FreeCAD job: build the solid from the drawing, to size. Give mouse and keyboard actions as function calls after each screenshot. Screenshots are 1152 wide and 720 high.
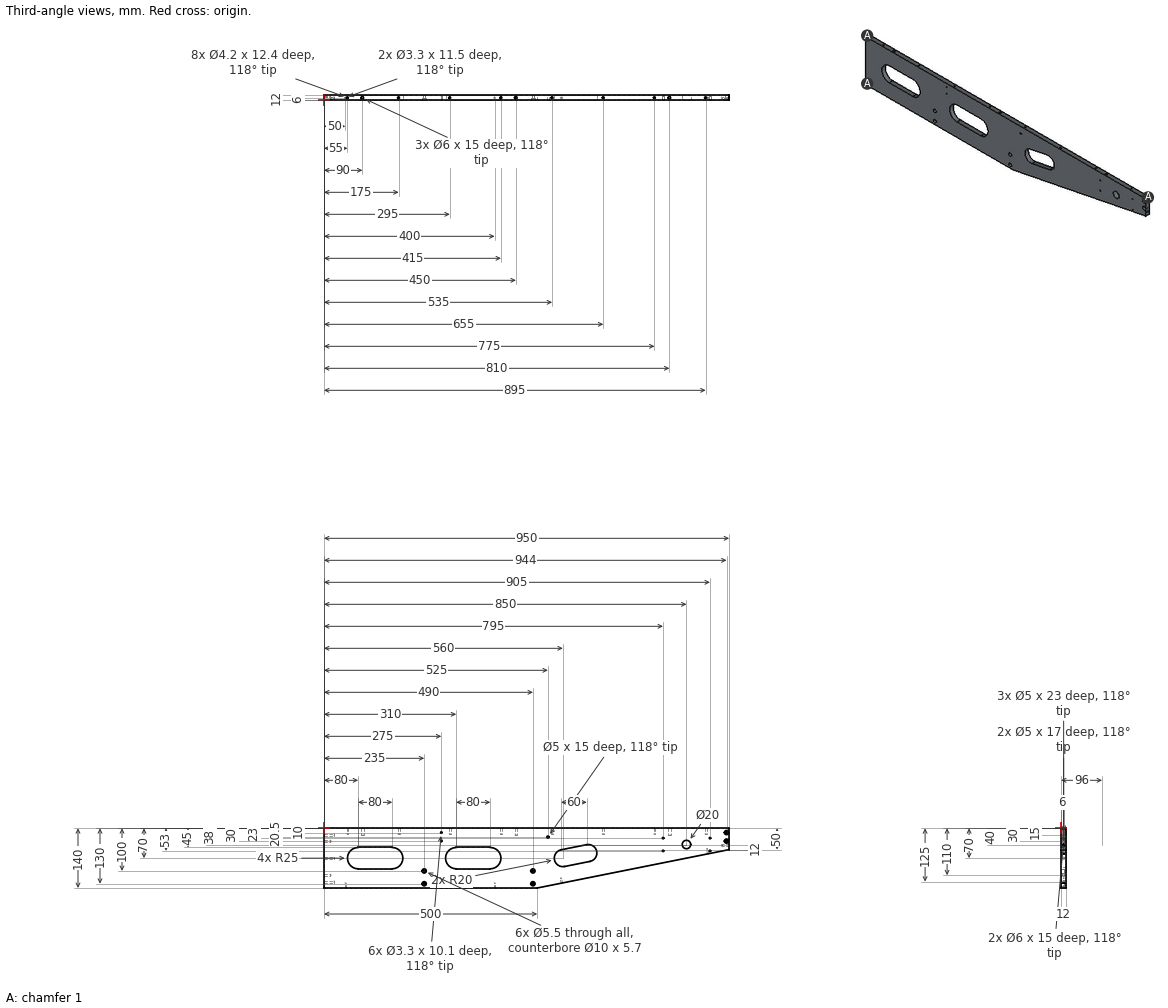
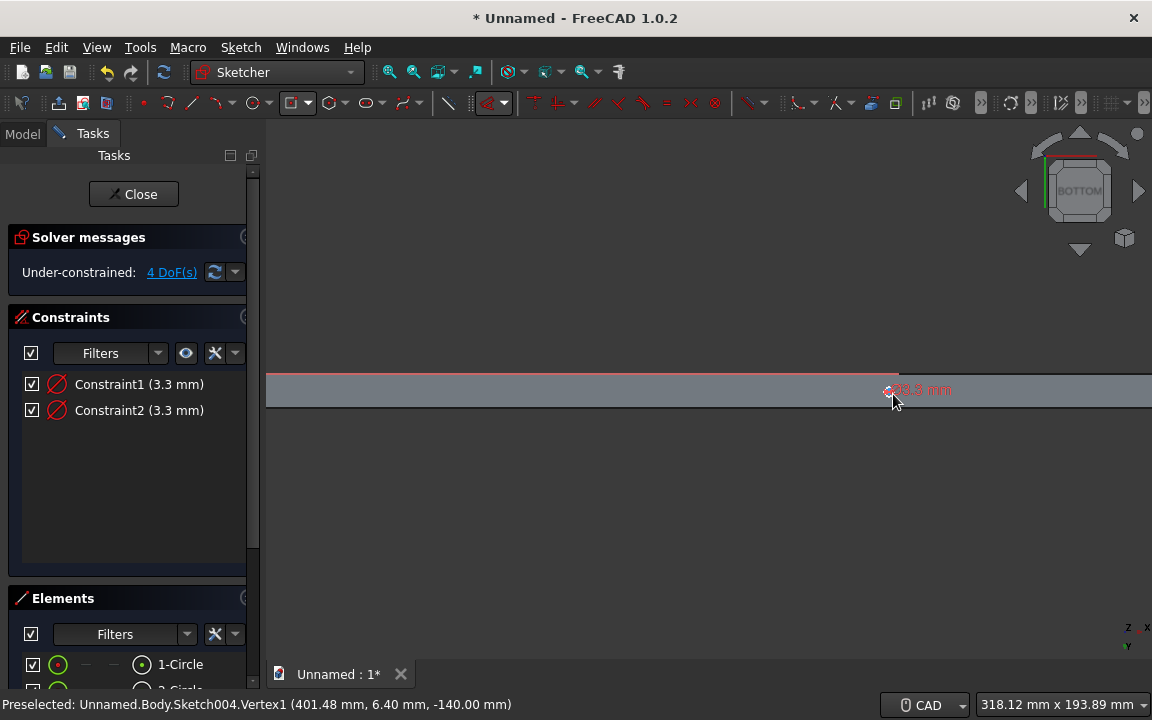
scroll(890, 392, down, 4)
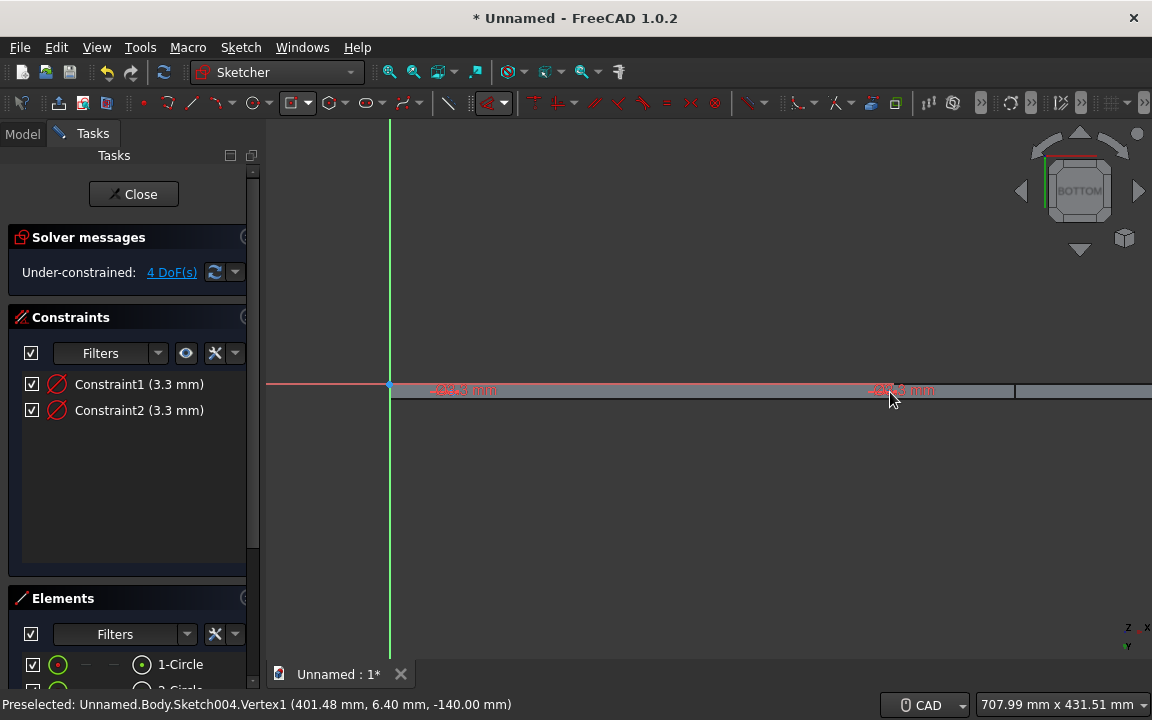
click(452, 392)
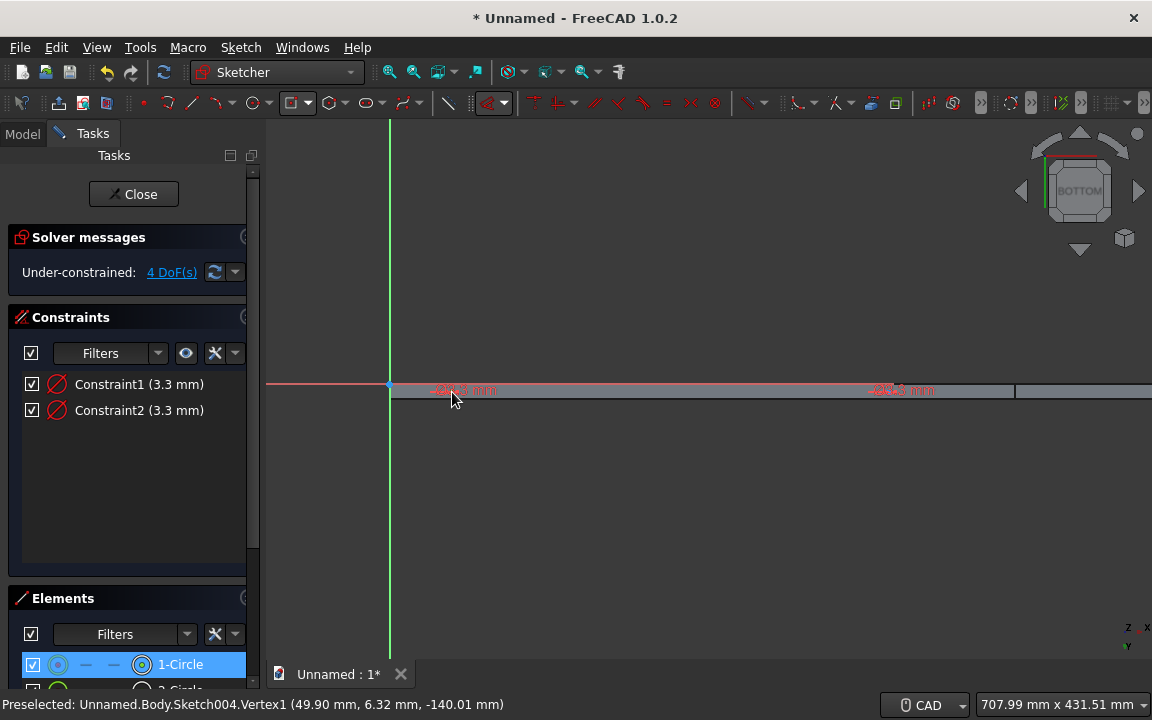
click(890, 392)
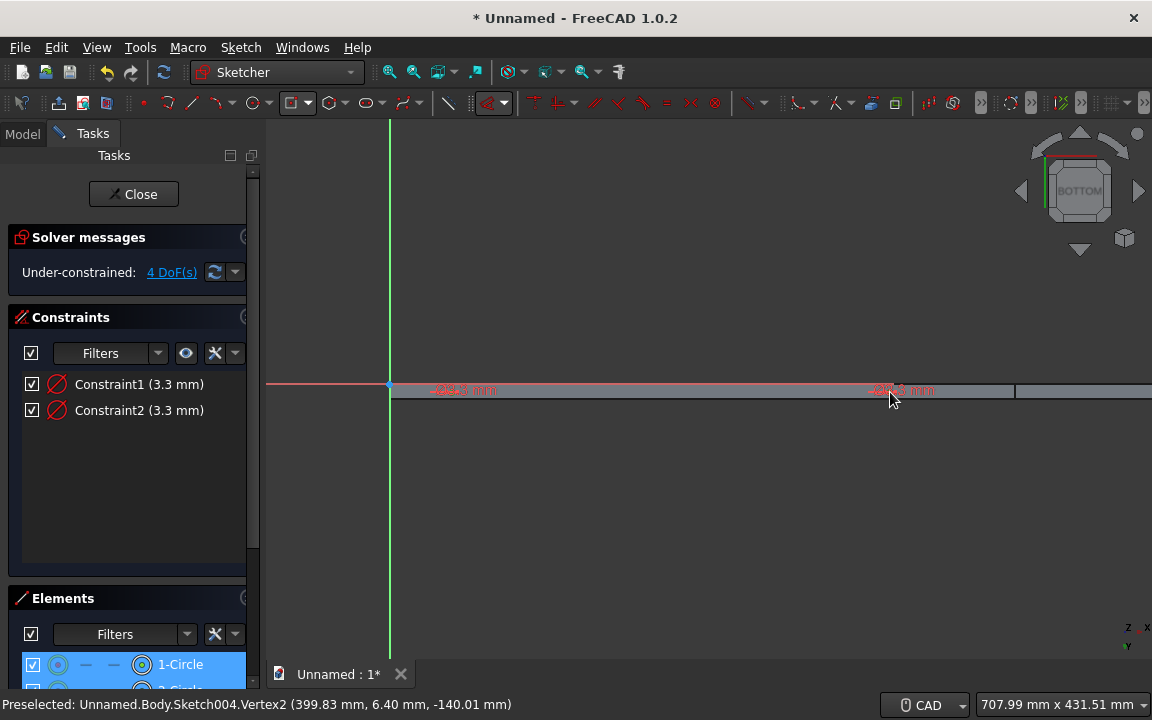
key(h)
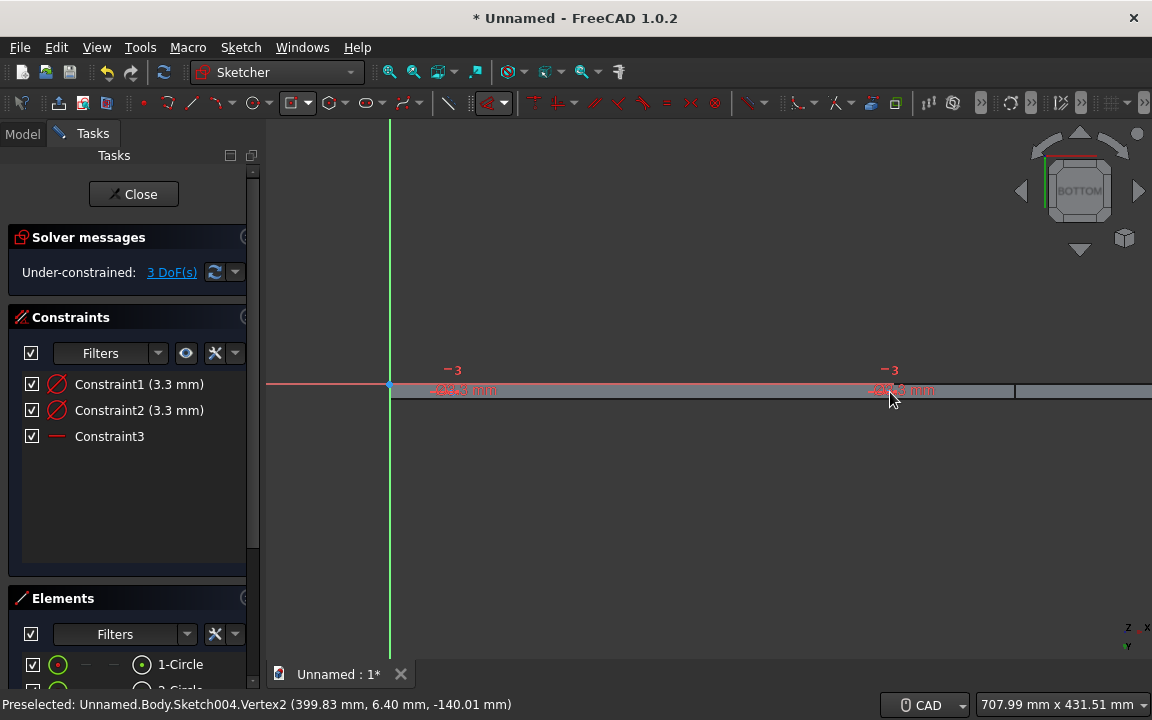
scroll(452, 392, up, 9)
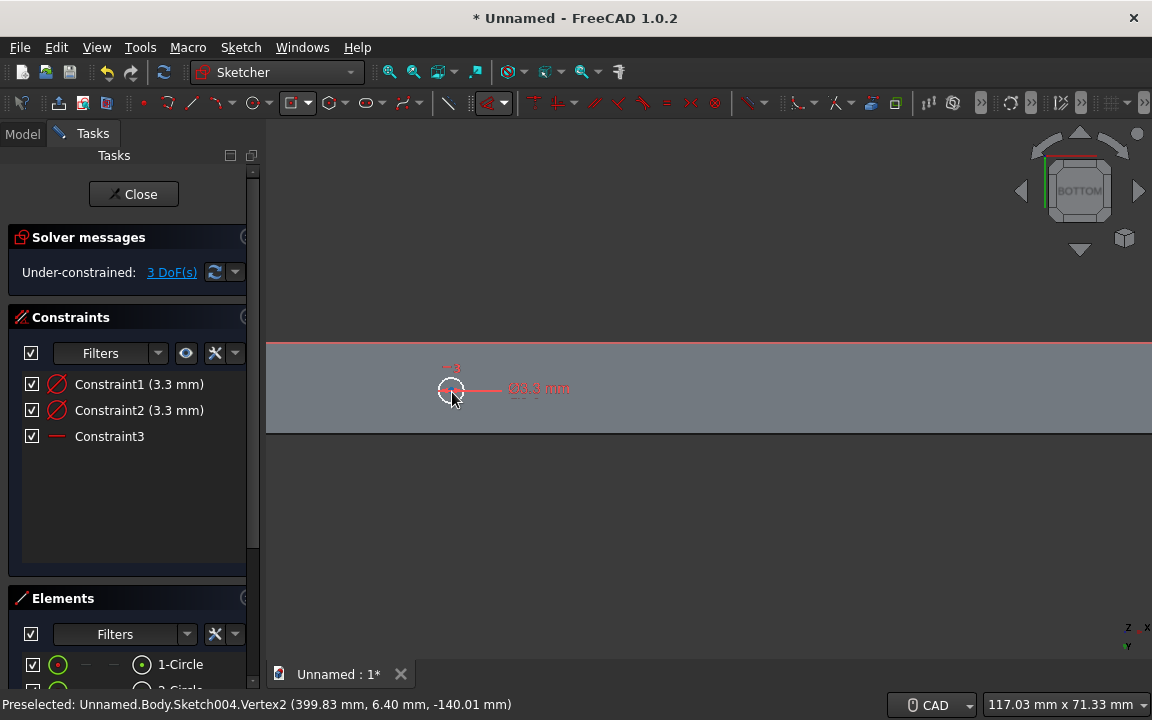
click(451, 391)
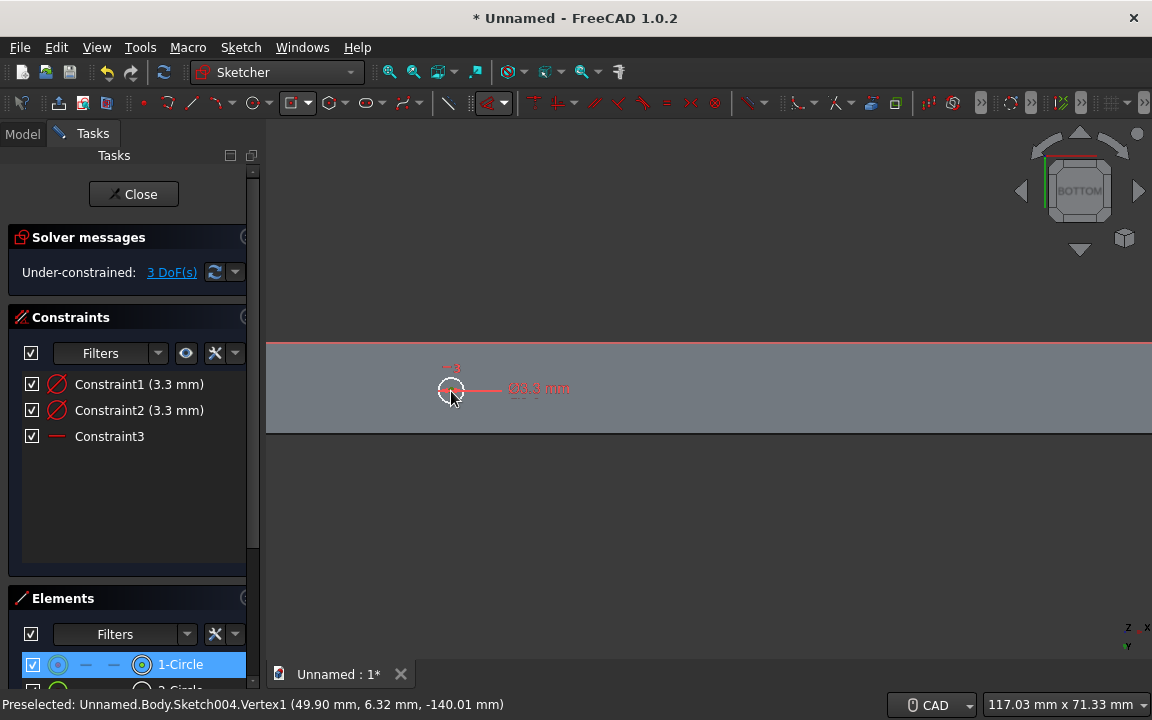
key(i)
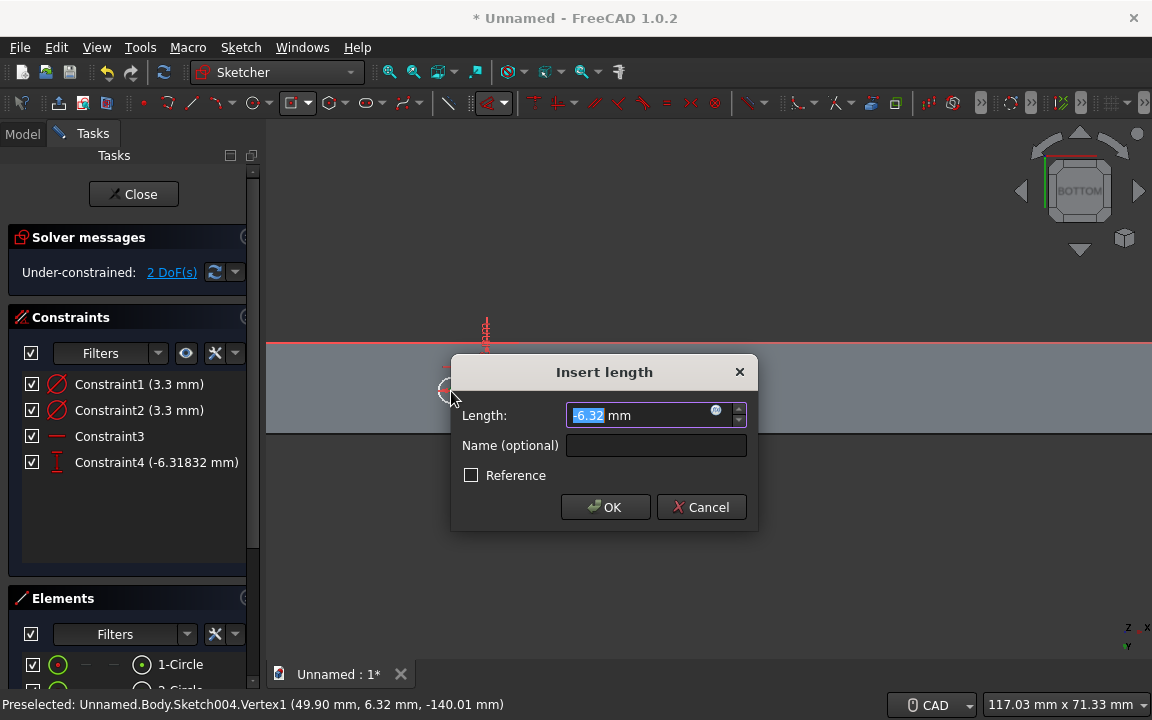
text(-6)
key(Return)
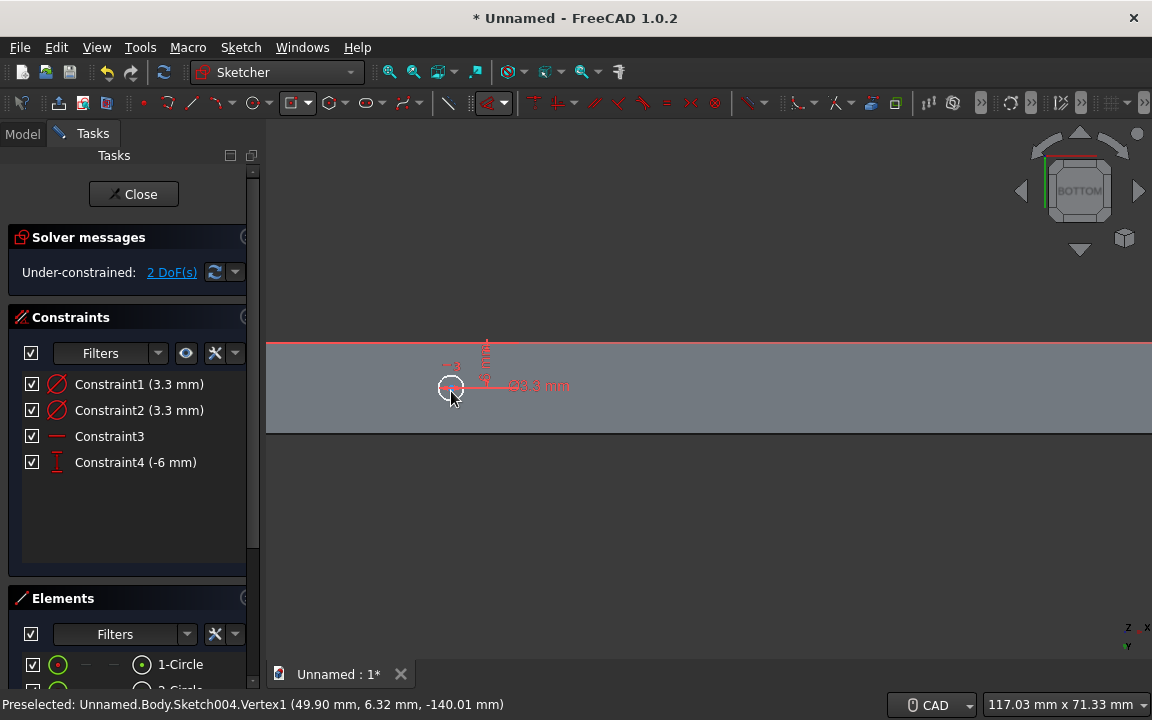
scroll(452, 392, down, 9)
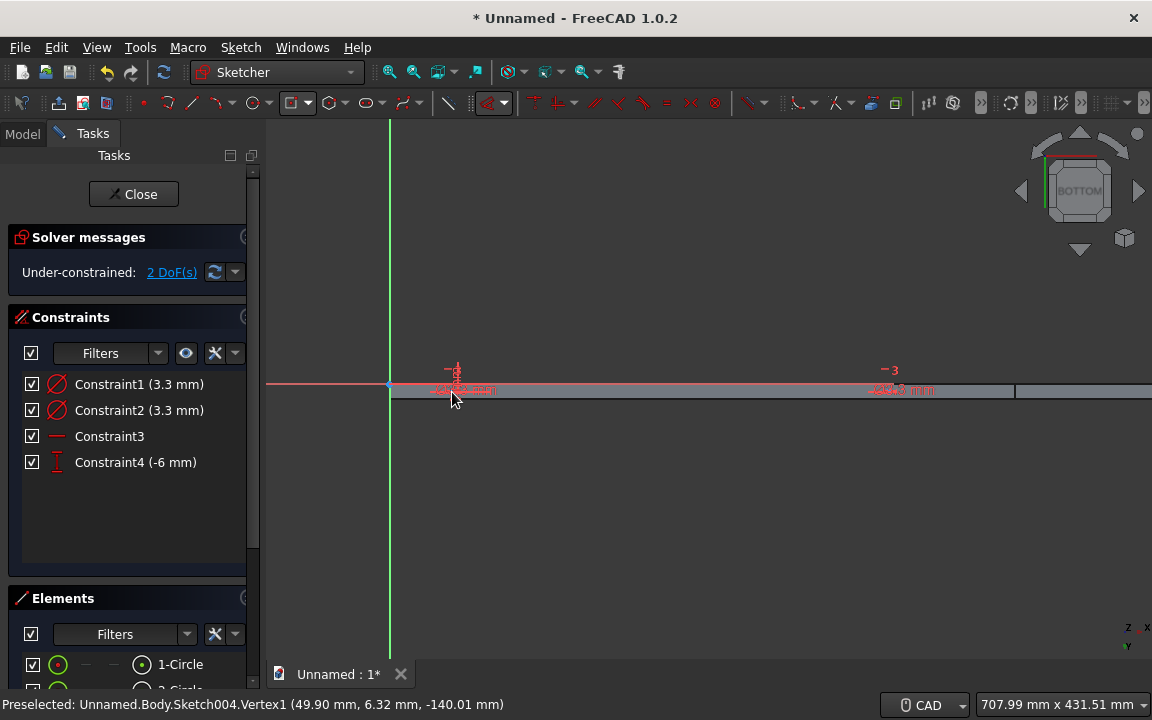
click(452, 392)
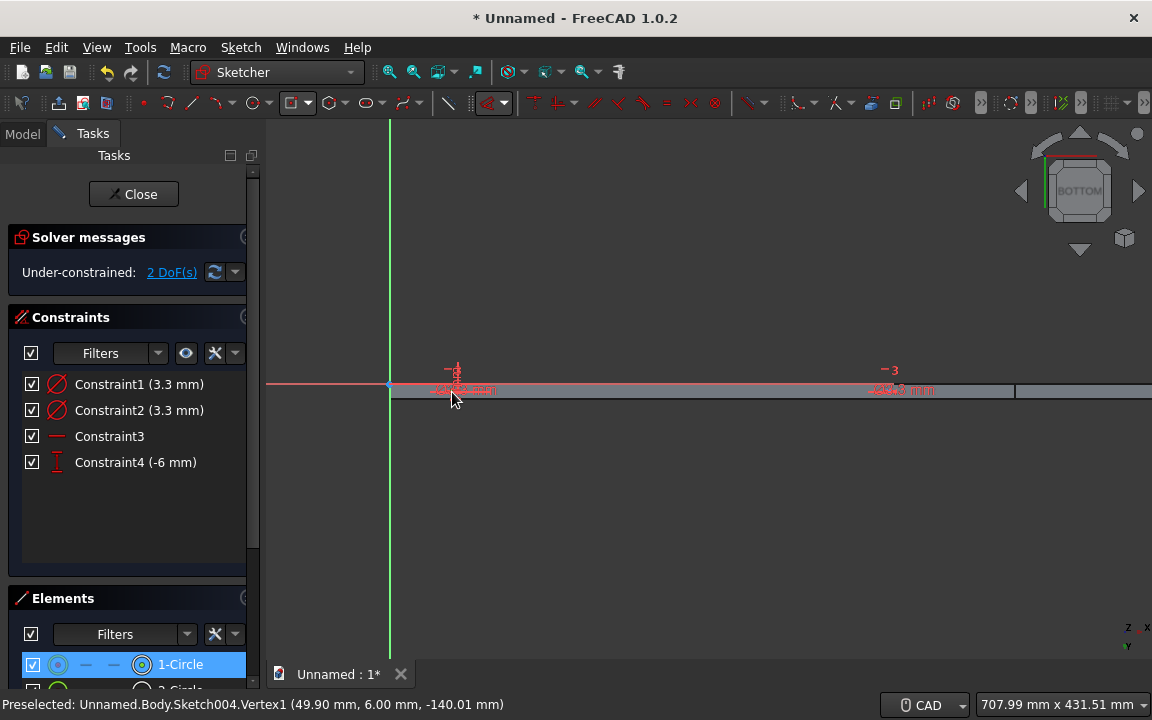
key(l)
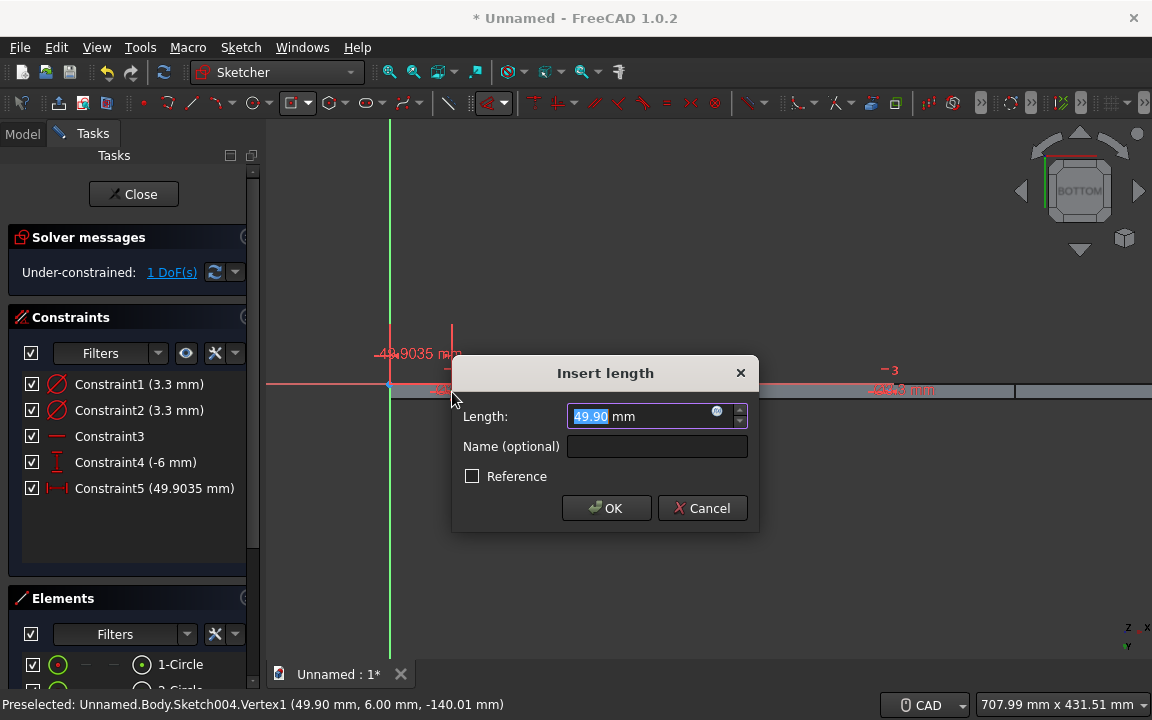
text(50)
key(Return)